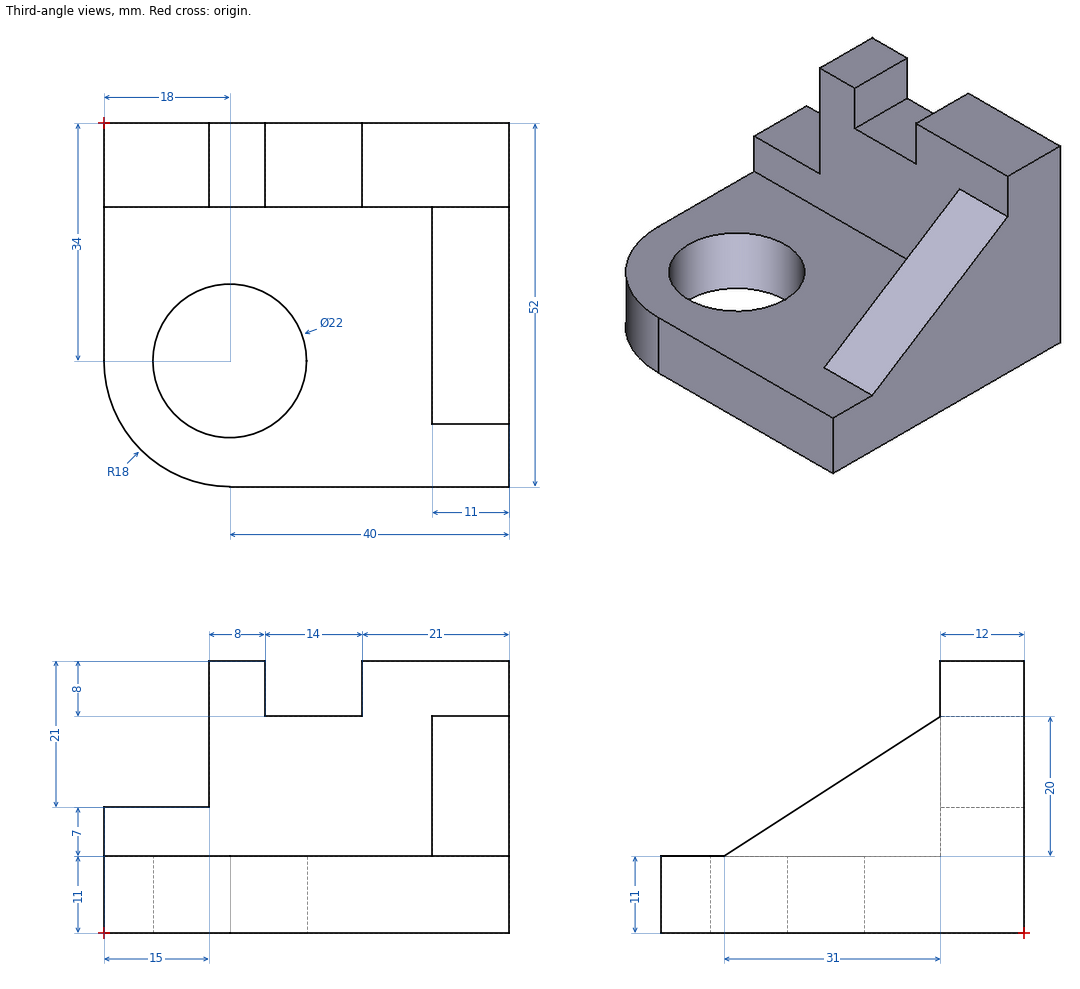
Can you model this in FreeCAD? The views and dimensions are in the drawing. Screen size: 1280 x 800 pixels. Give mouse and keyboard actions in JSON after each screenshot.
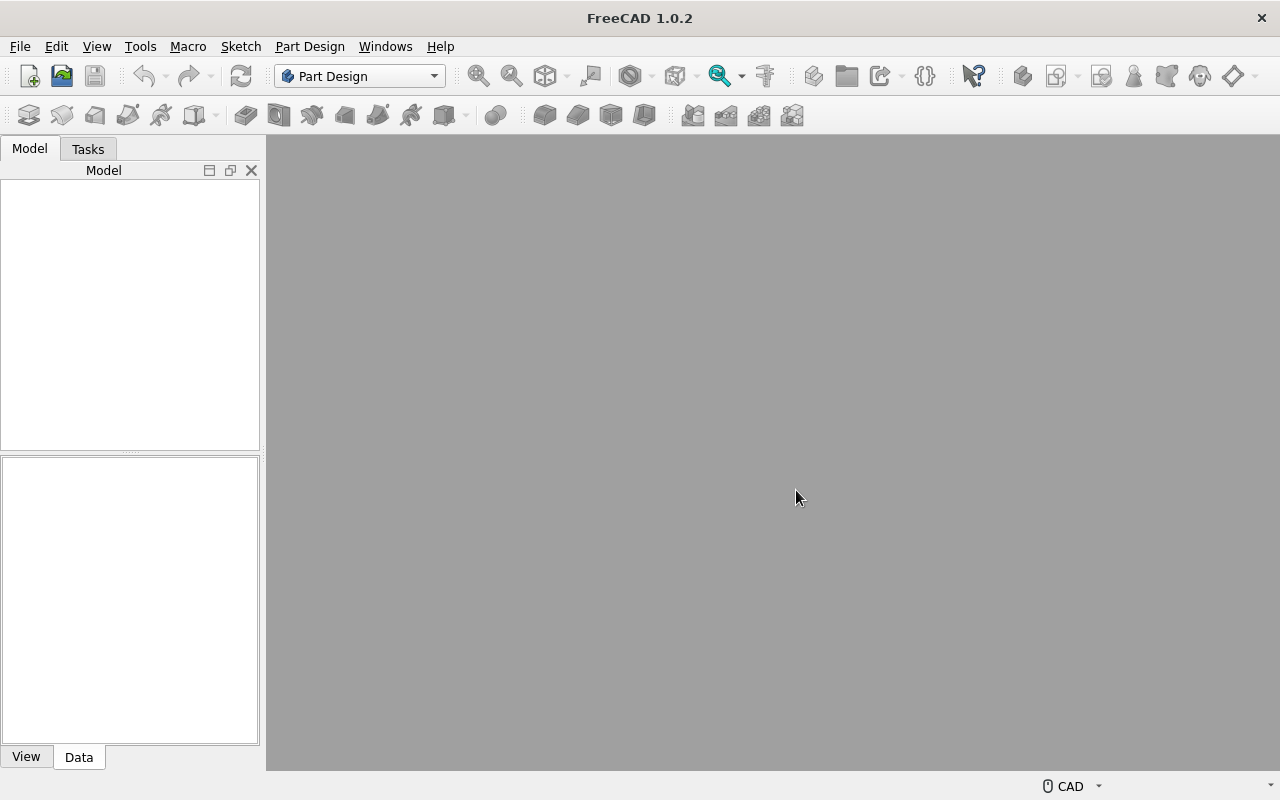
{"action": "left_click", "coordinate": [29, 76]}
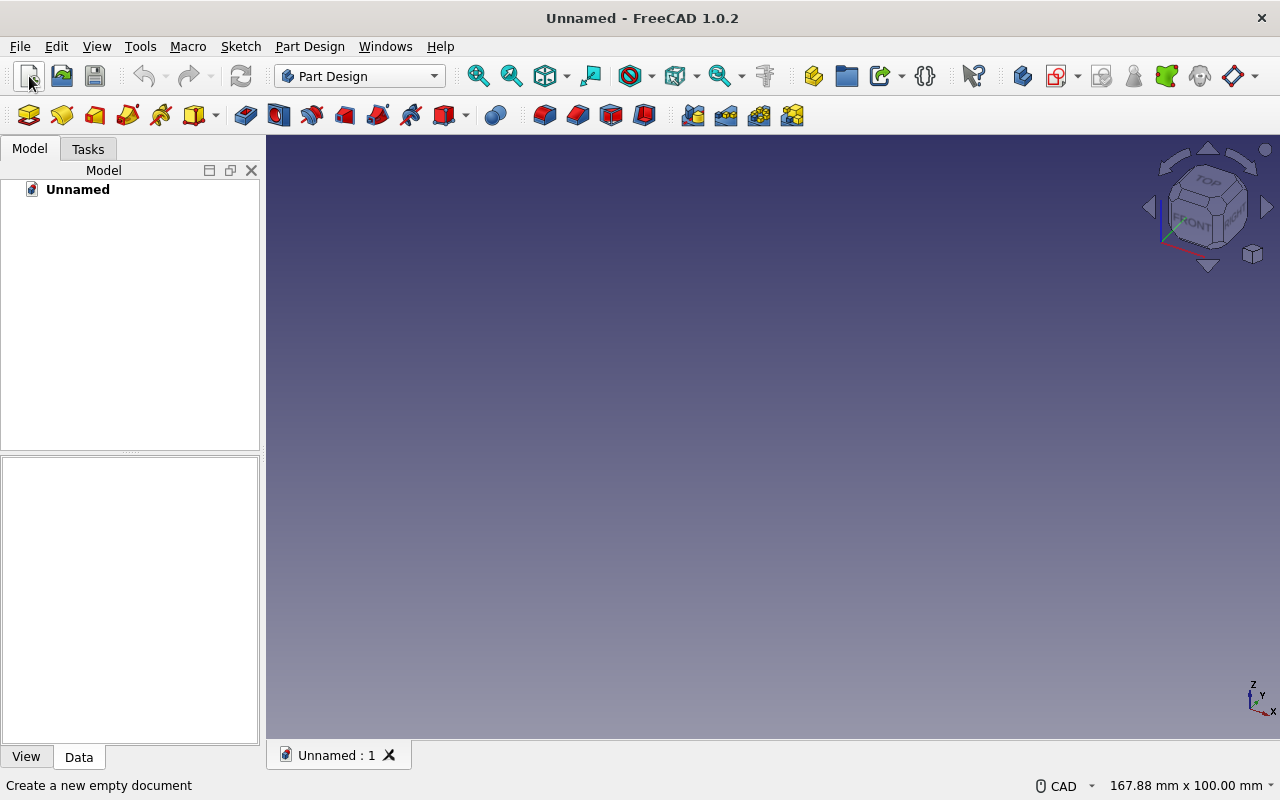
{"action": "left_click", "coordinate": [1056, 76]}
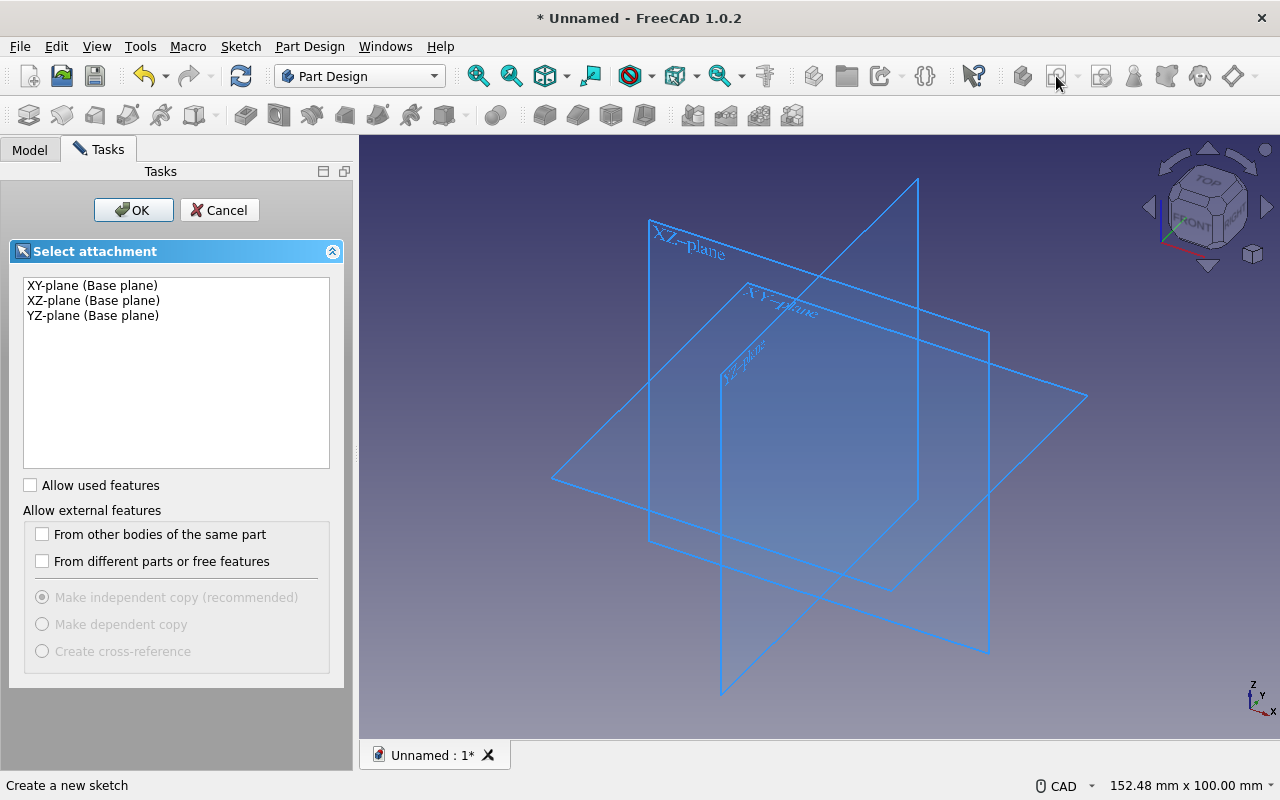
{"action": "left_click", "coordinate": [84, 286]}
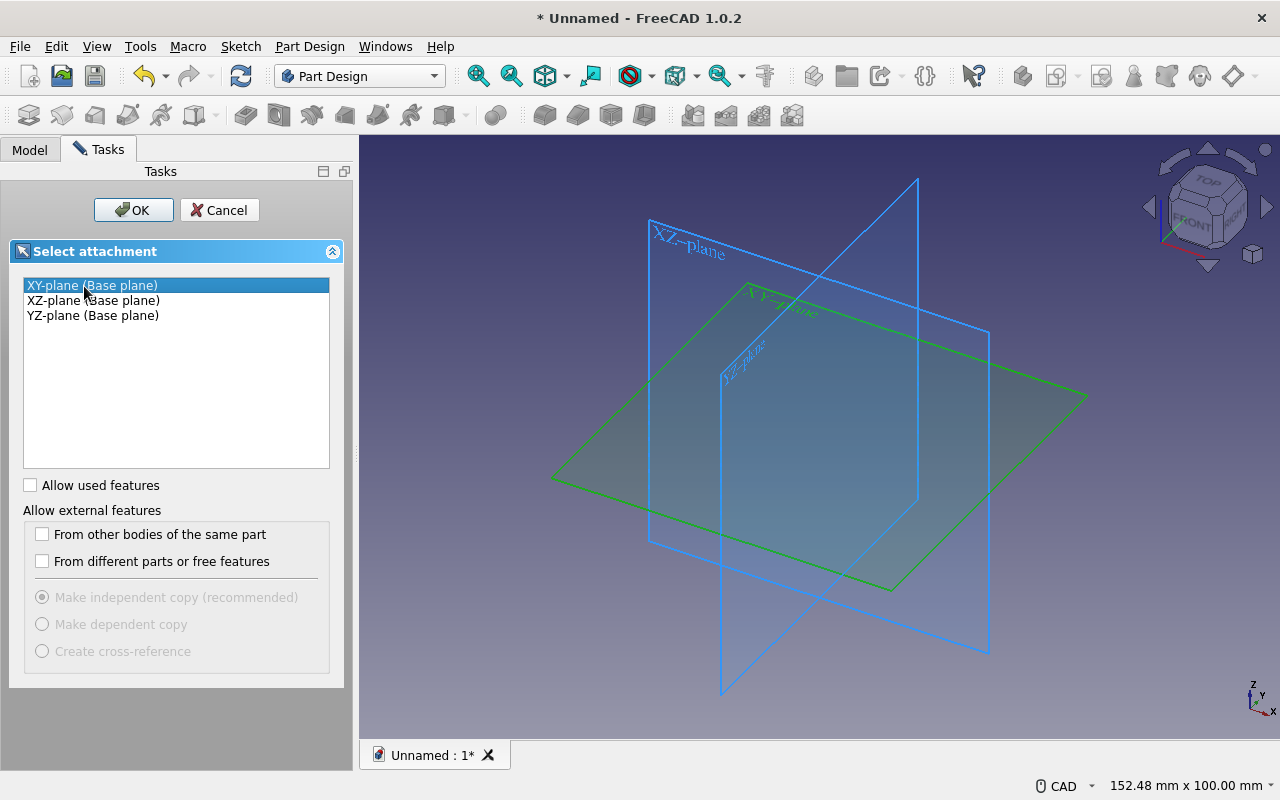
{"action": "left_click", "coordinate": [134, 210]}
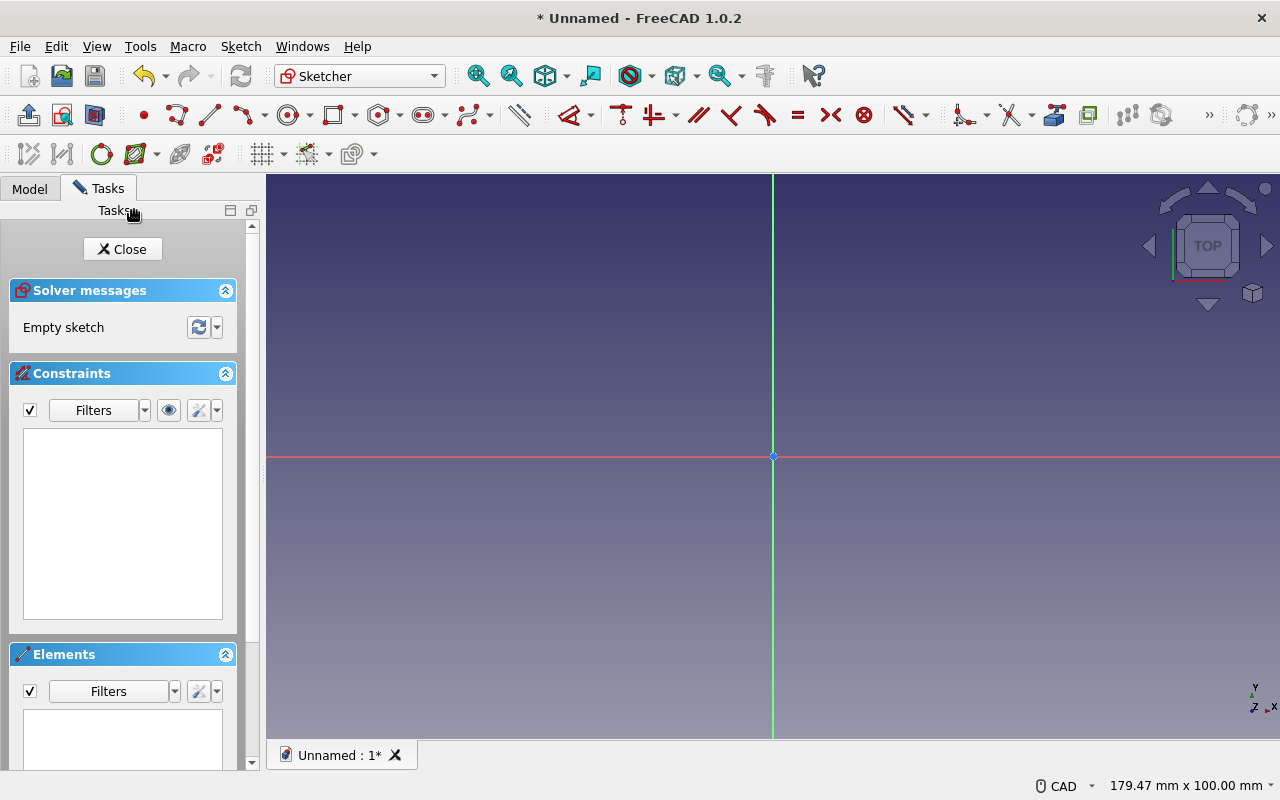
{"action": "scroll", "coordinate": [294, 202], "scroll_direction": "down", "scroll_amount": 1}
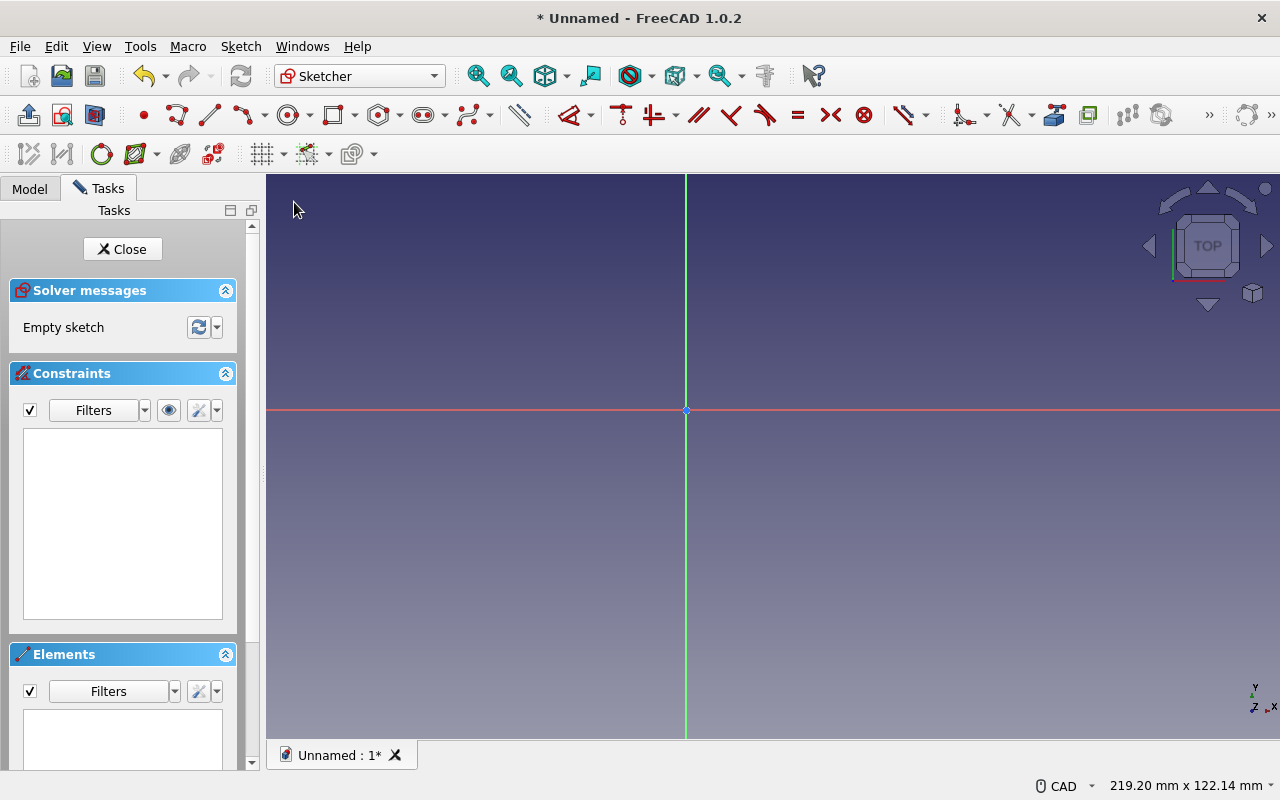
{"action": "scroll", "coordinate": [1056, 681], "scroll_direction": "up", "scroll_amount": 2}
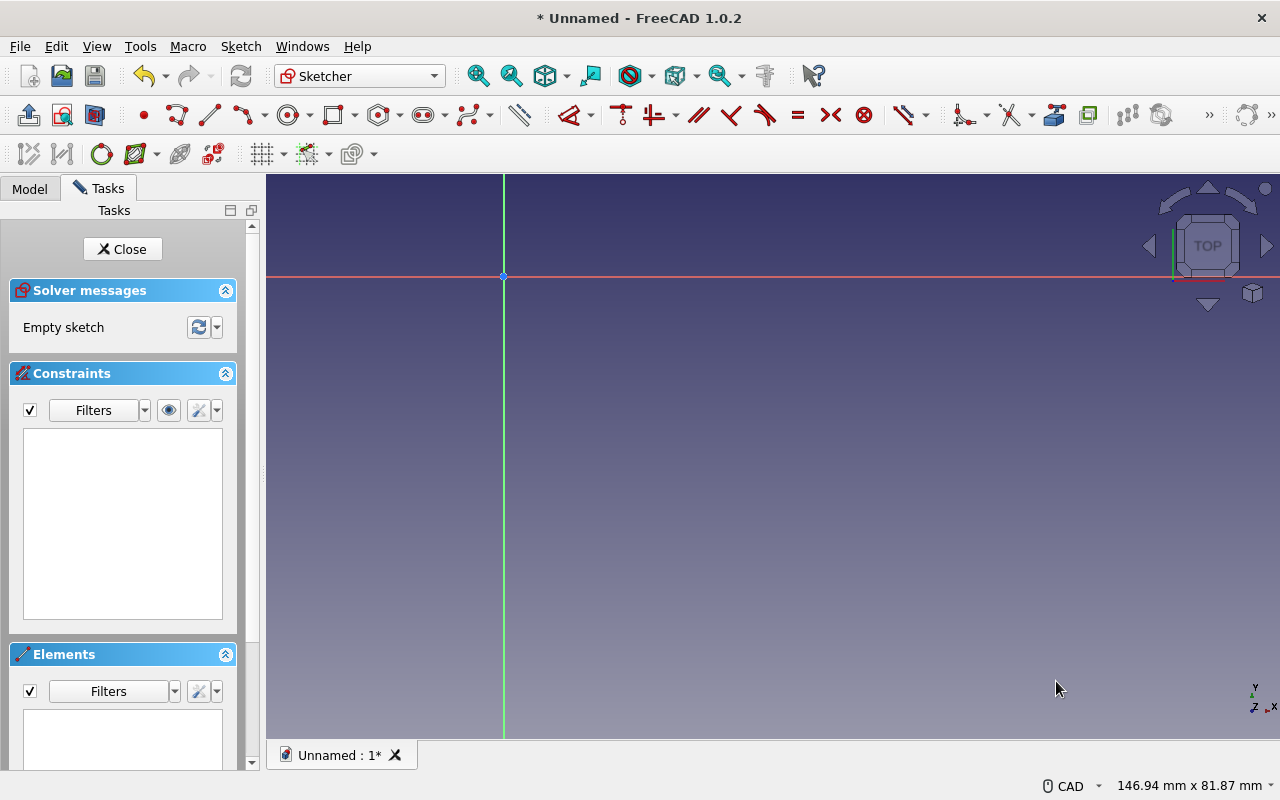
{"action": "left_click", "coordinate": [177, 116]}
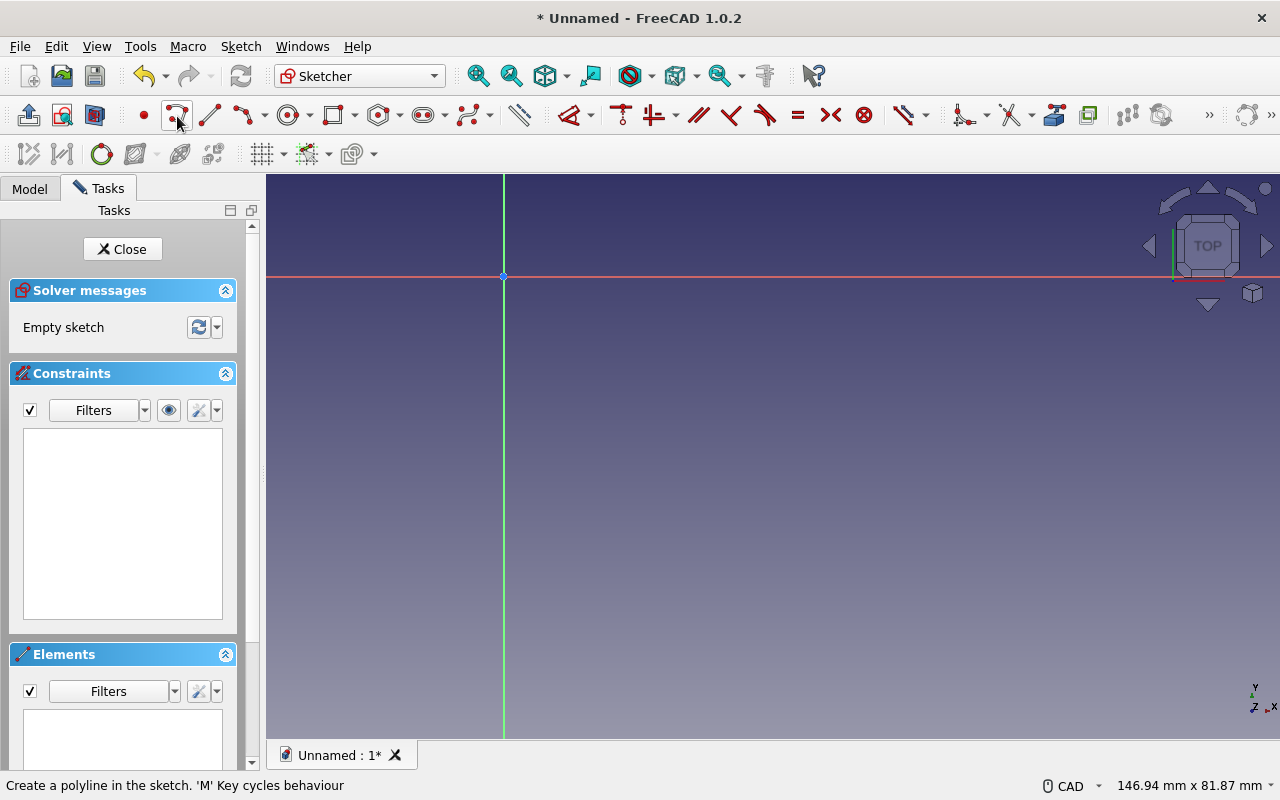
{"action": "left_click", "coordinate": [628, 636]}
{"action": "left_click", "coordinate": [904, 636]}
{"action": "left_click", "coordinate": [904, 277]}
{"action": "left_click", "coordinate": [504, 277]}
{"action": "left_click", "coordinate": [513, 511]}
{"action": "right_click", "coordinate": [513, 511]}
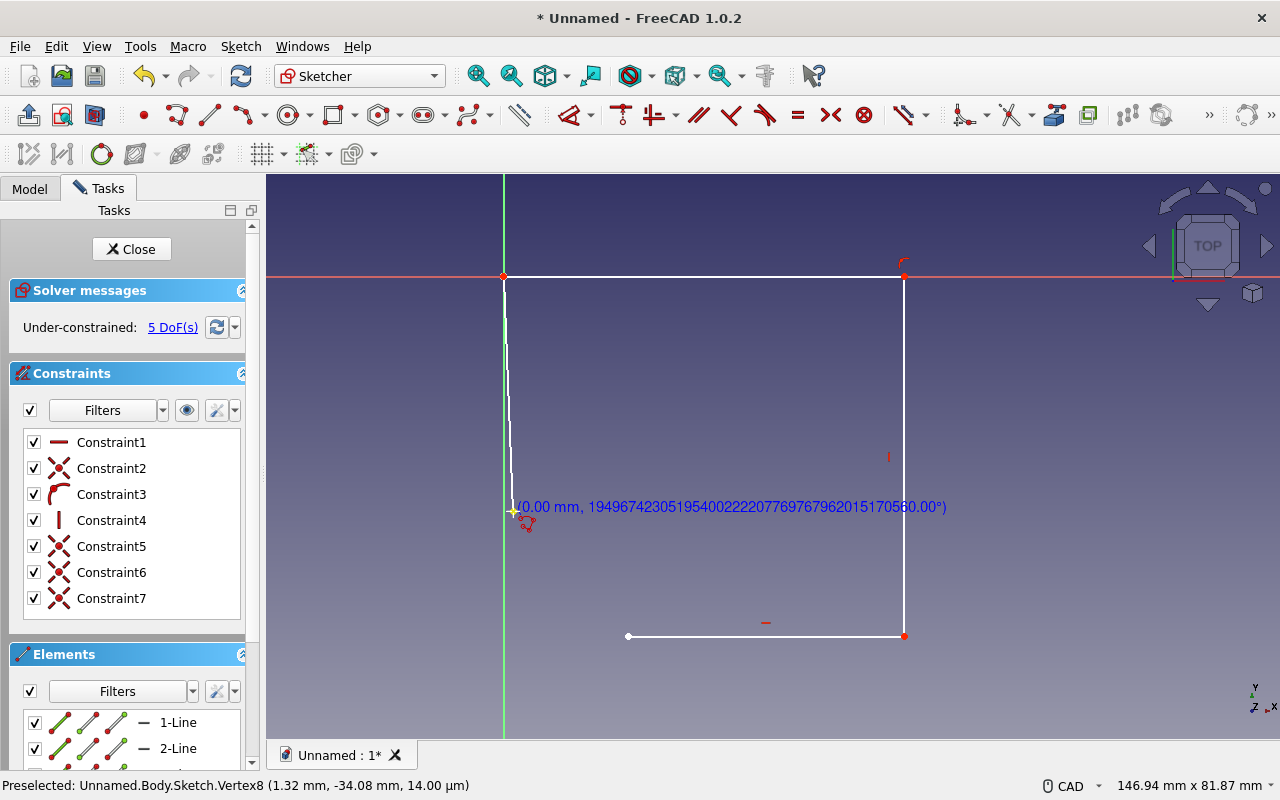
{"action": "left_click", "coordinate": [242, 116]}